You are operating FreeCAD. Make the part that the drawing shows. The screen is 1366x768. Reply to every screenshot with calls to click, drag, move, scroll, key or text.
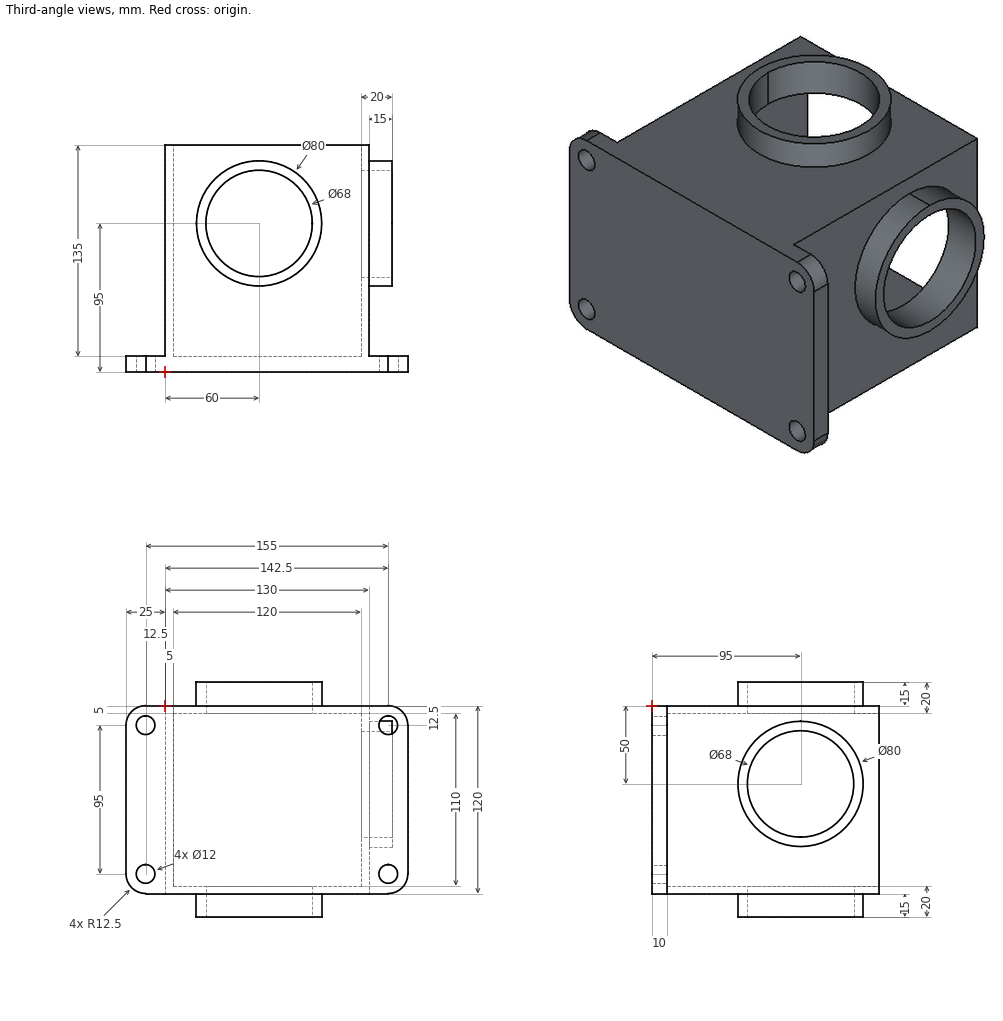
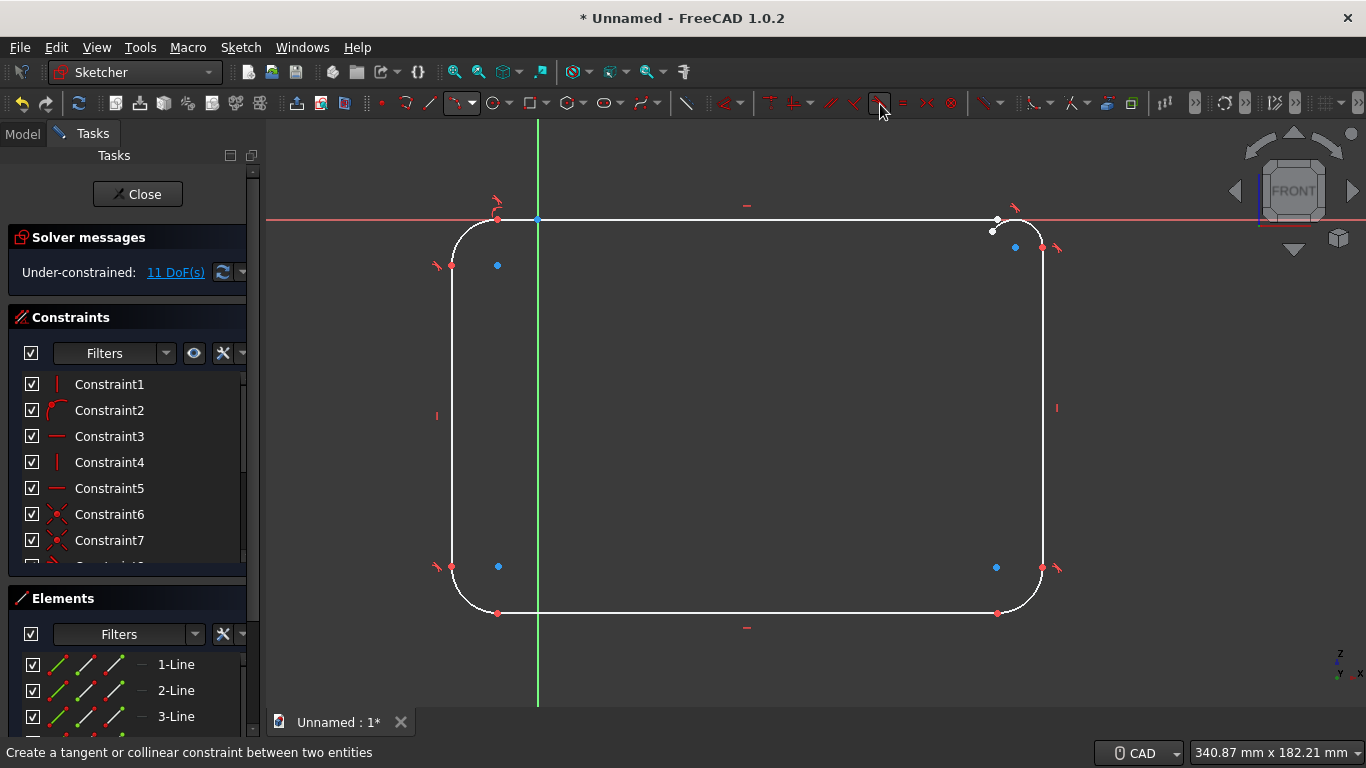
click(847, 613)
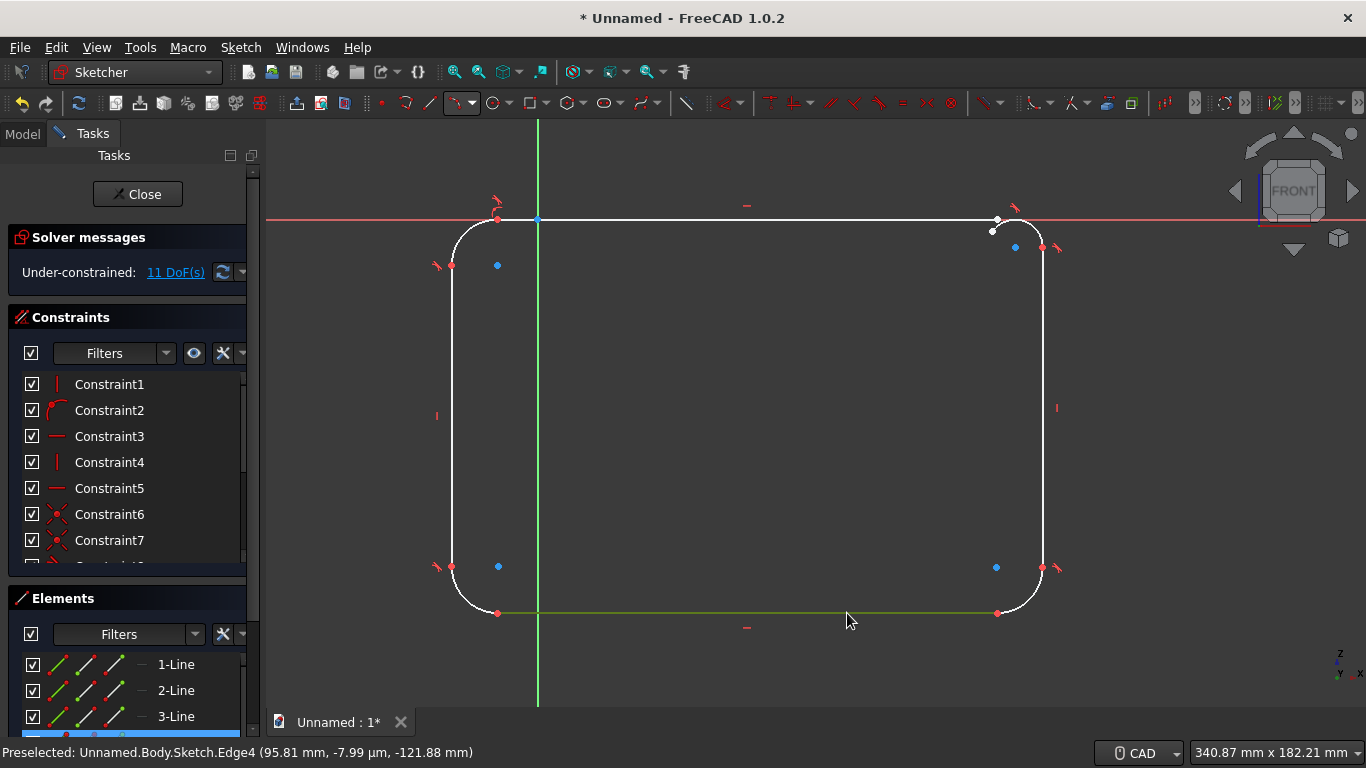
click(1018, 608)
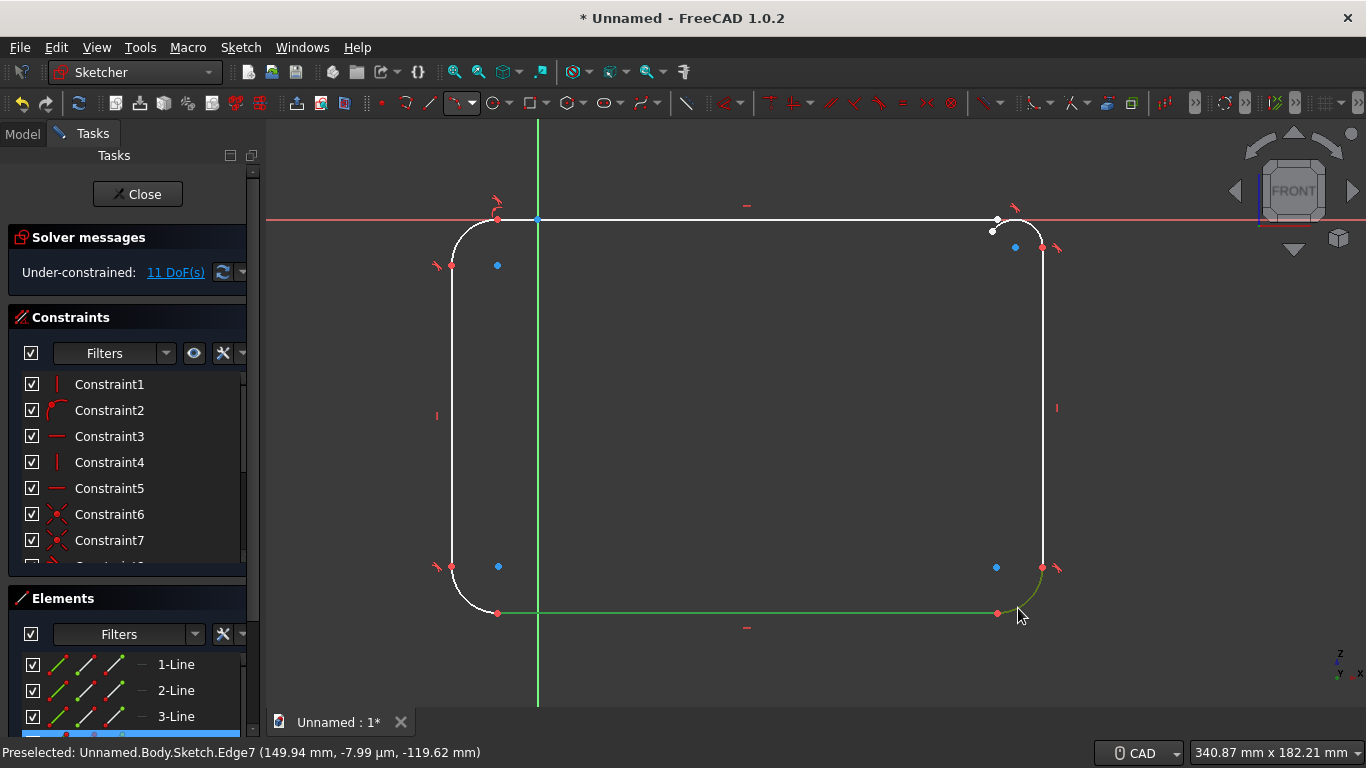
click(880, 104)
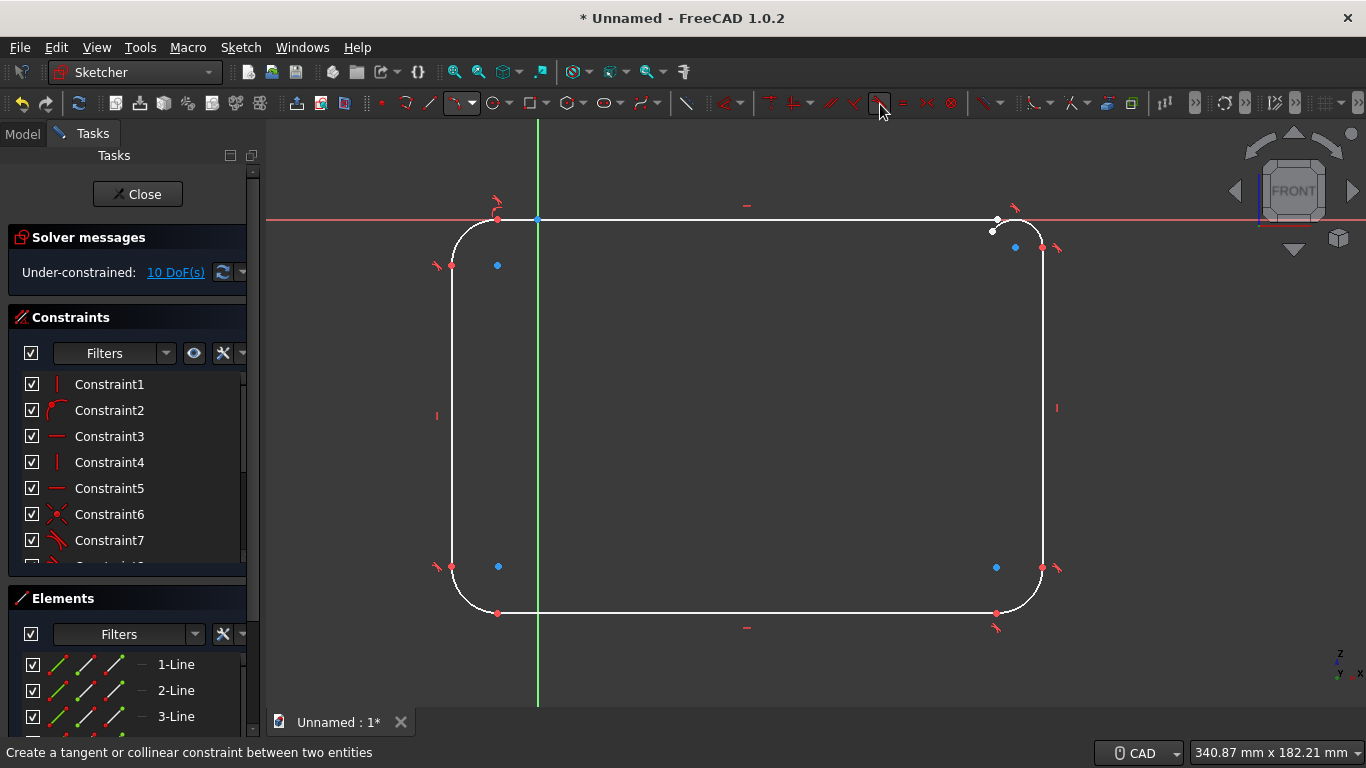
click(847, 613)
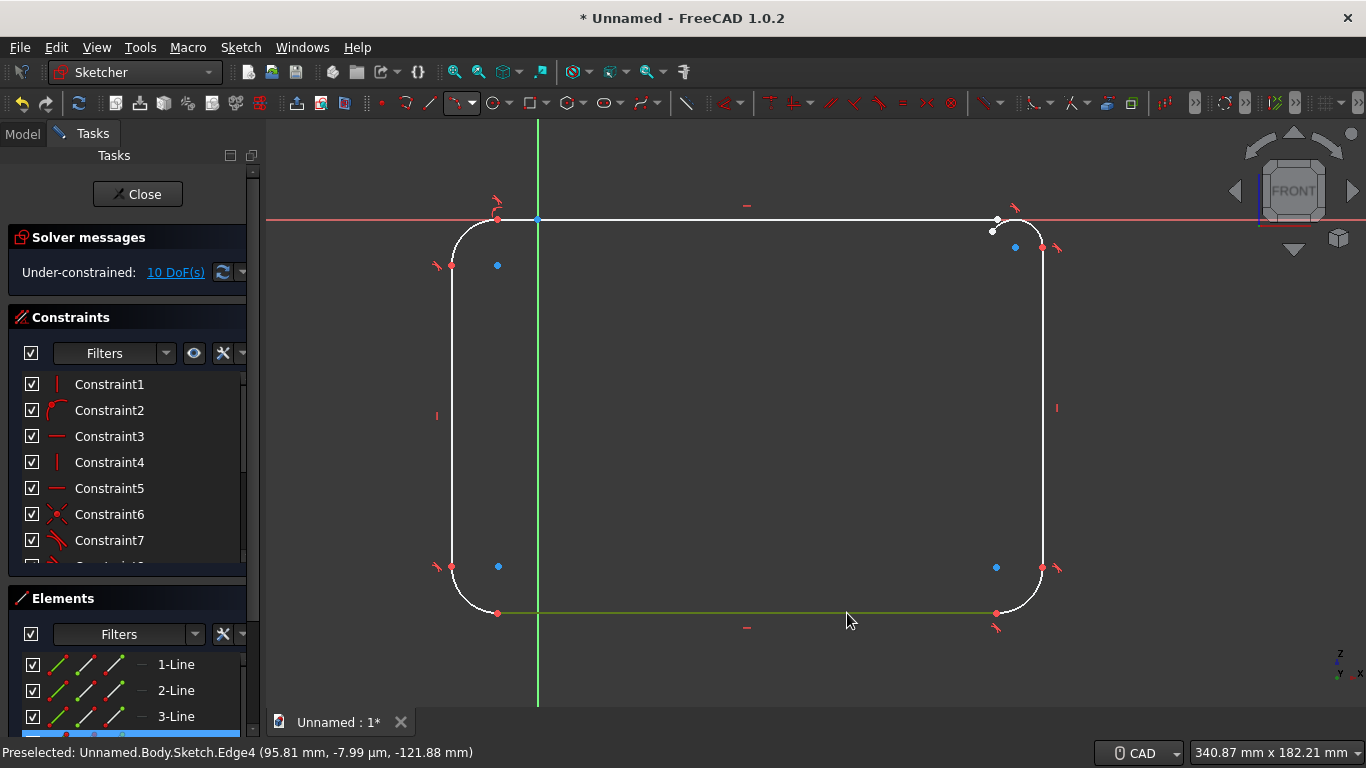
click(457, 587)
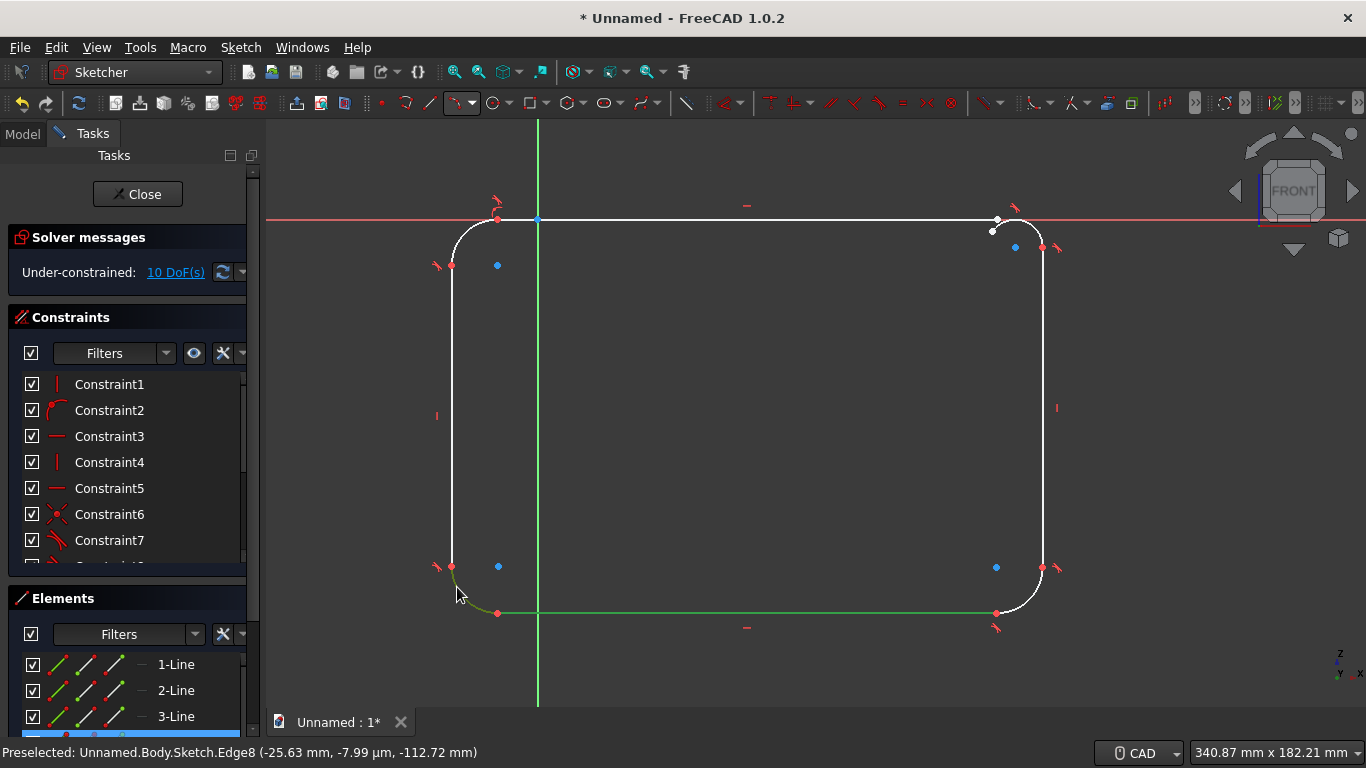
click(880, 104)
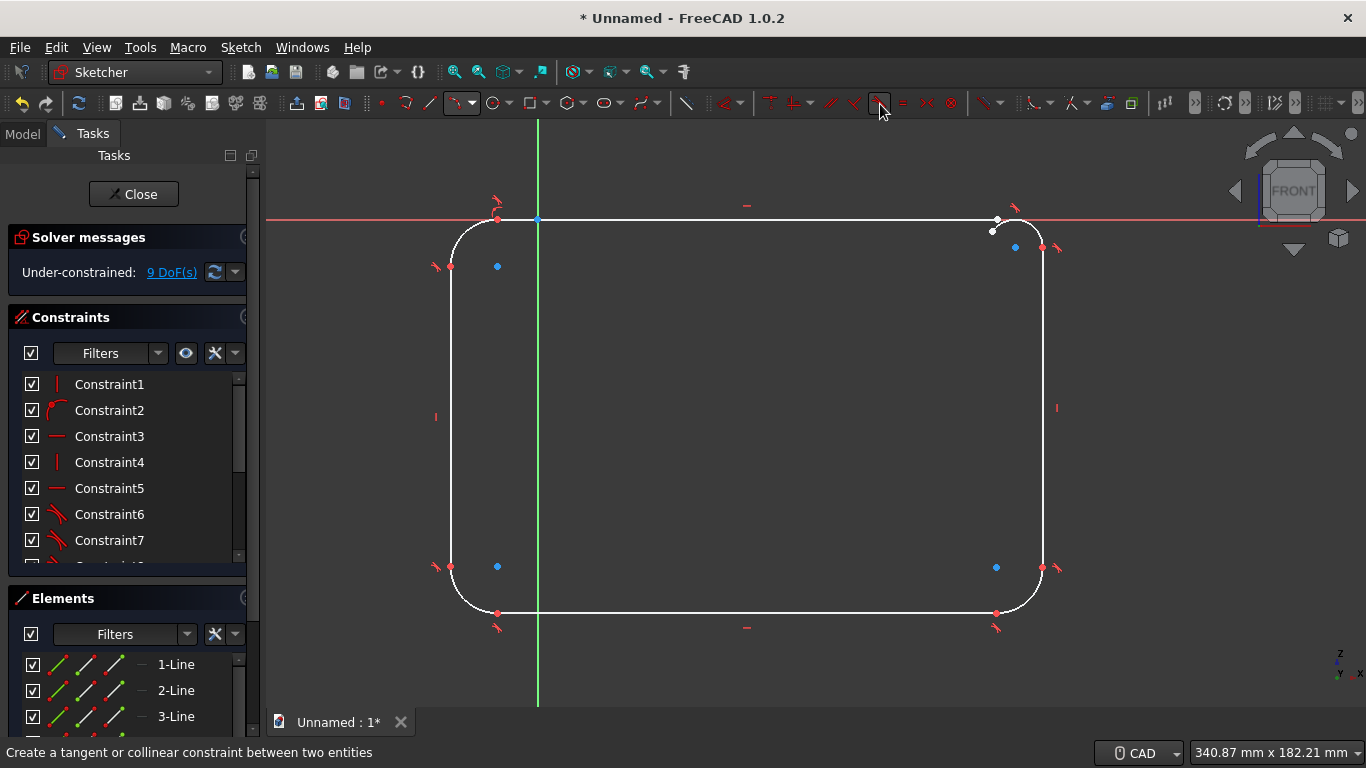
click(456, 245)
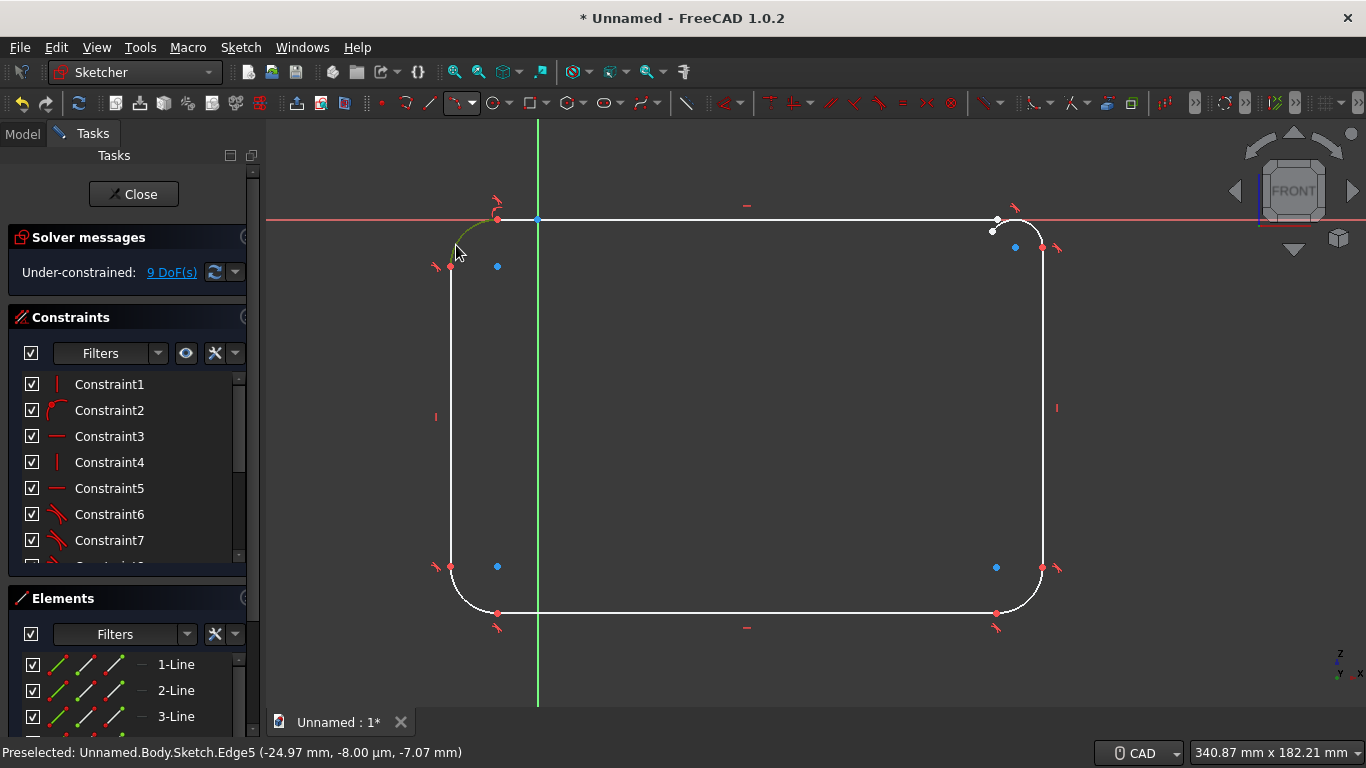
click(1009, 220)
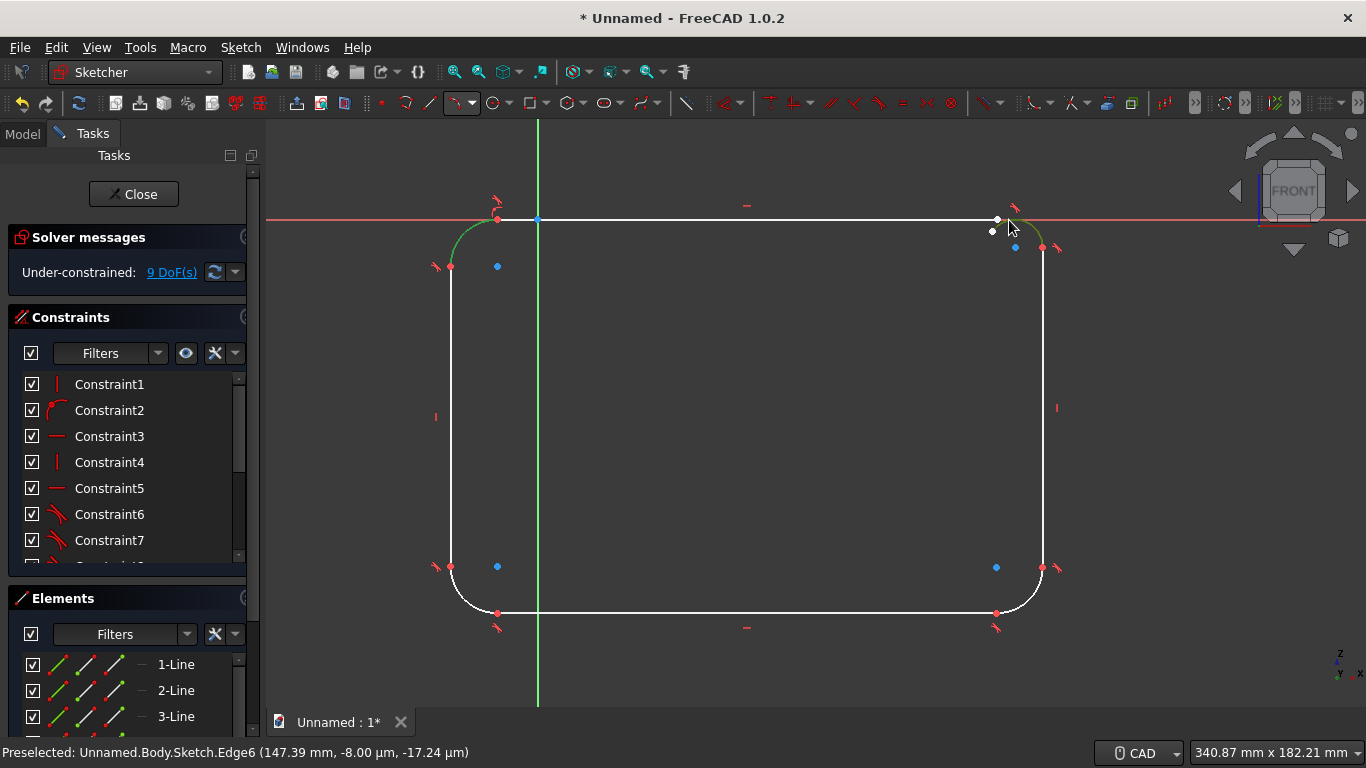
click(1018, 608)